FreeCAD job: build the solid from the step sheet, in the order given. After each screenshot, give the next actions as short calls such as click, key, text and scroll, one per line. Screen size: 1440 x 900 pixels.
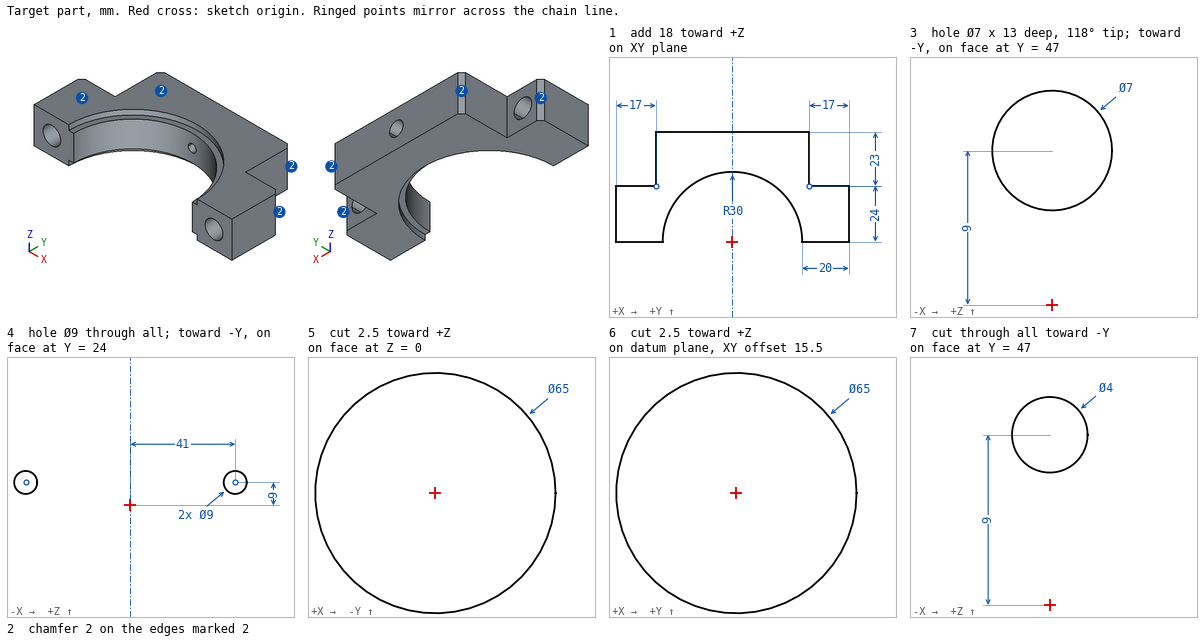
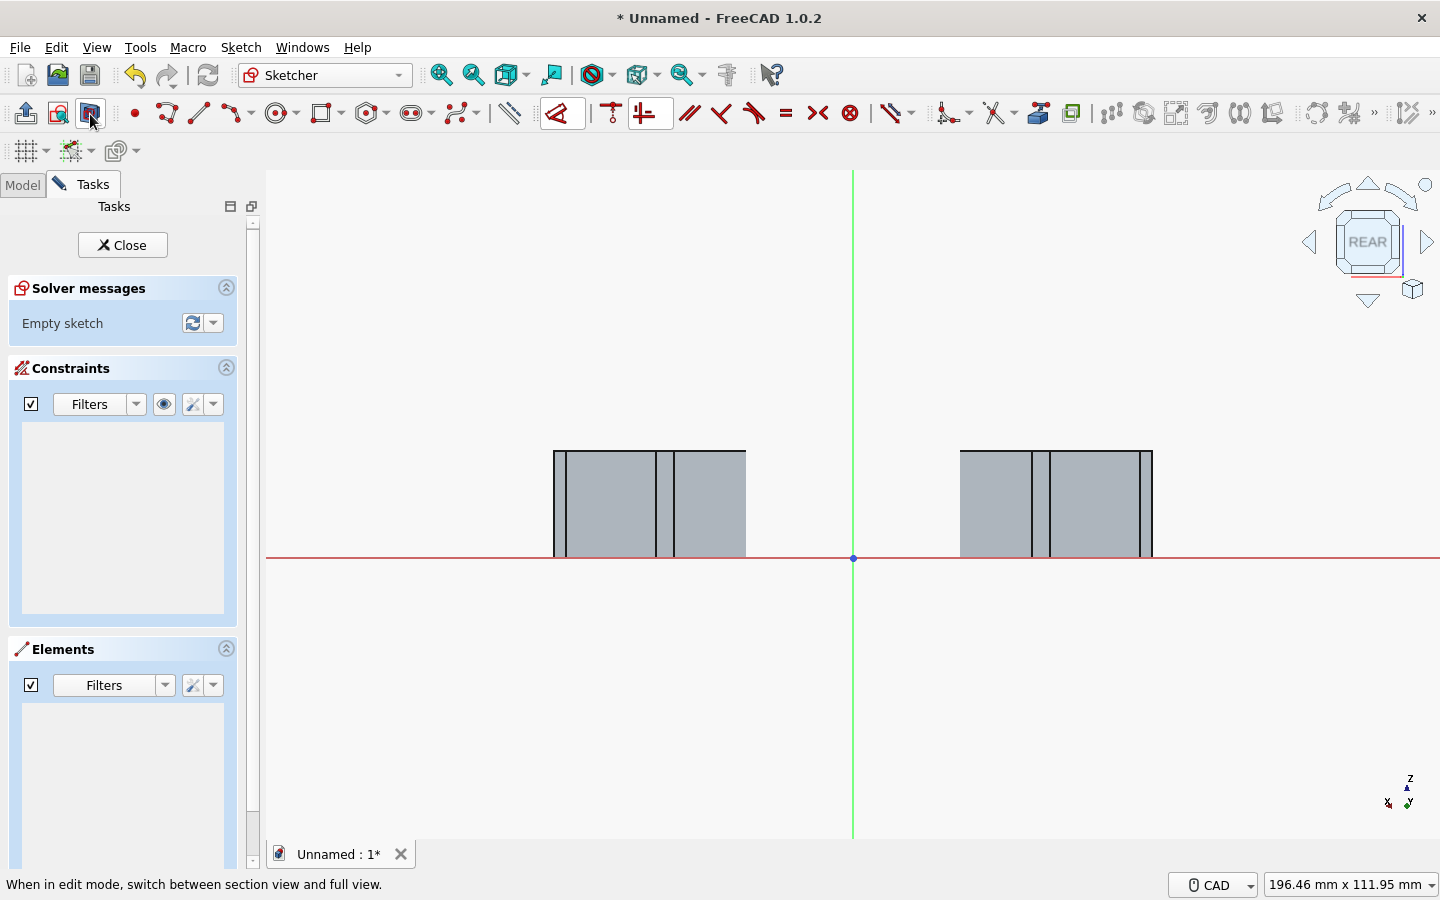
click(276, 114)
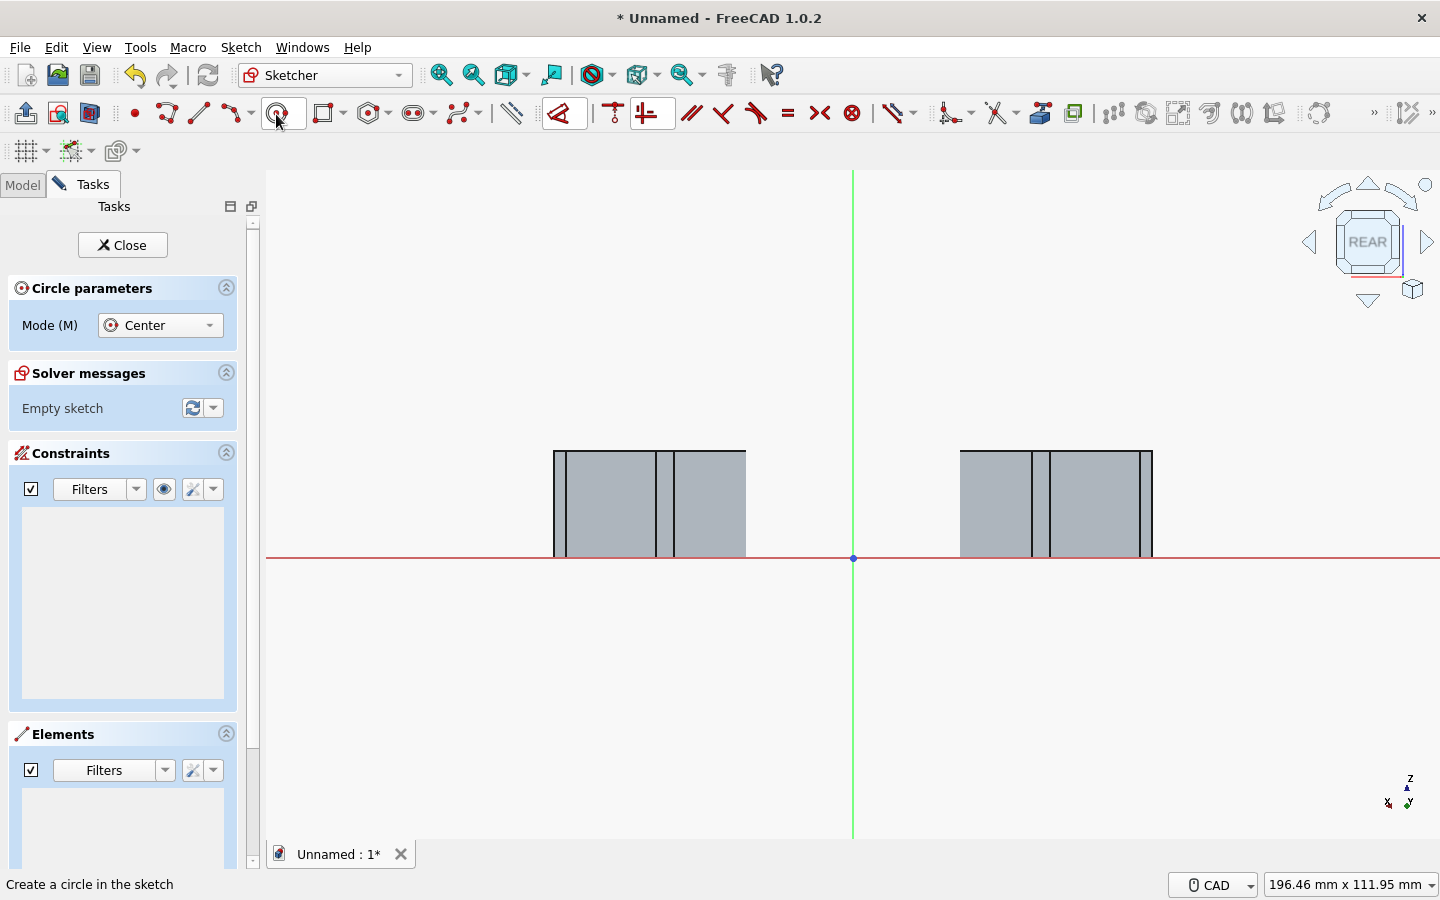
click(1098, 505)
click(1117, 485)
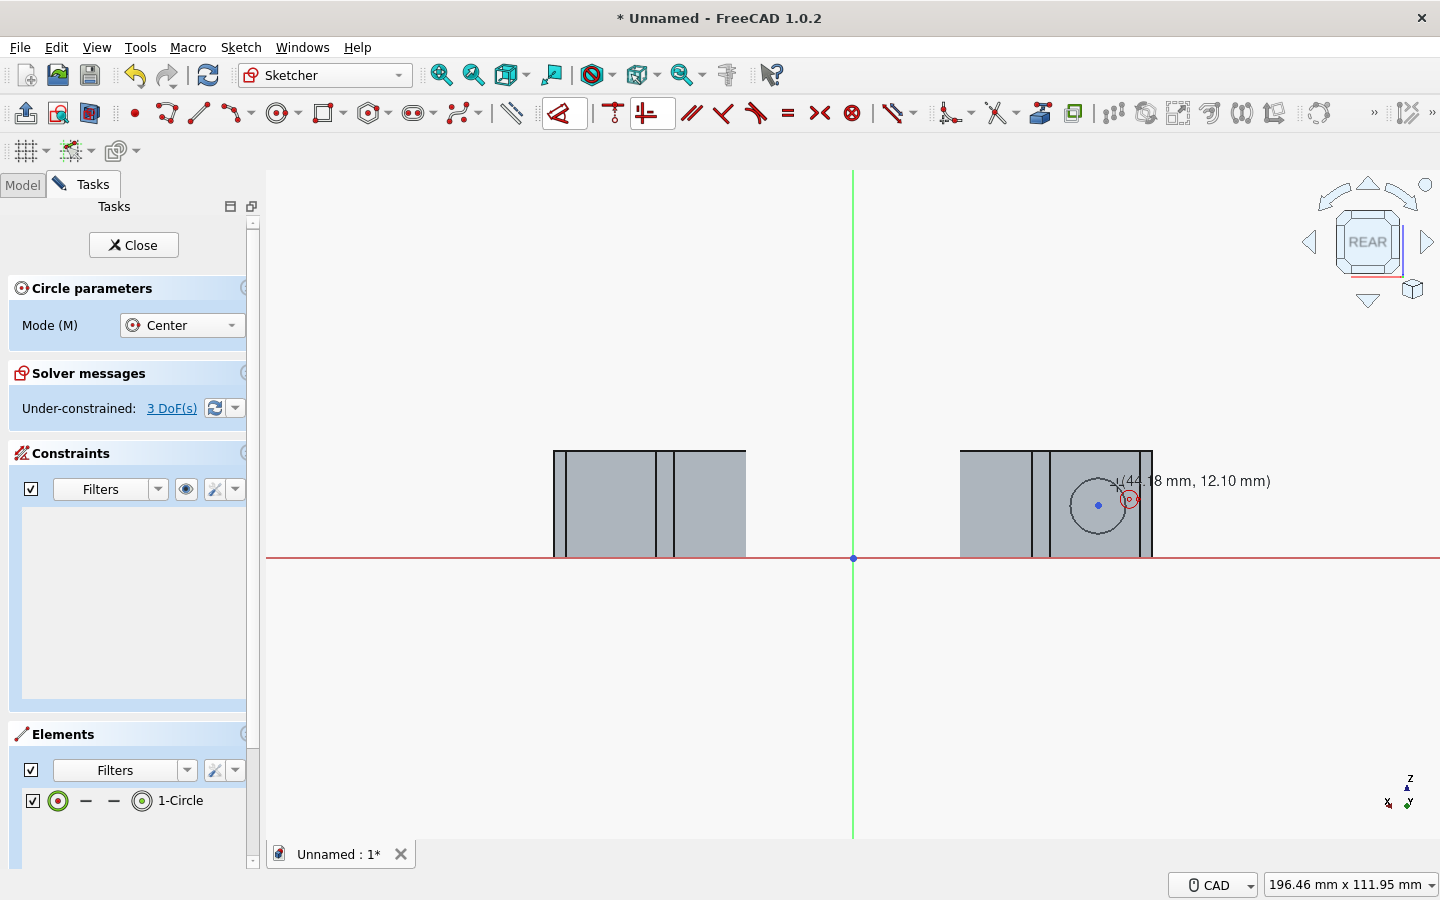
click(608, 505)
click(627, 485)
key(Escape)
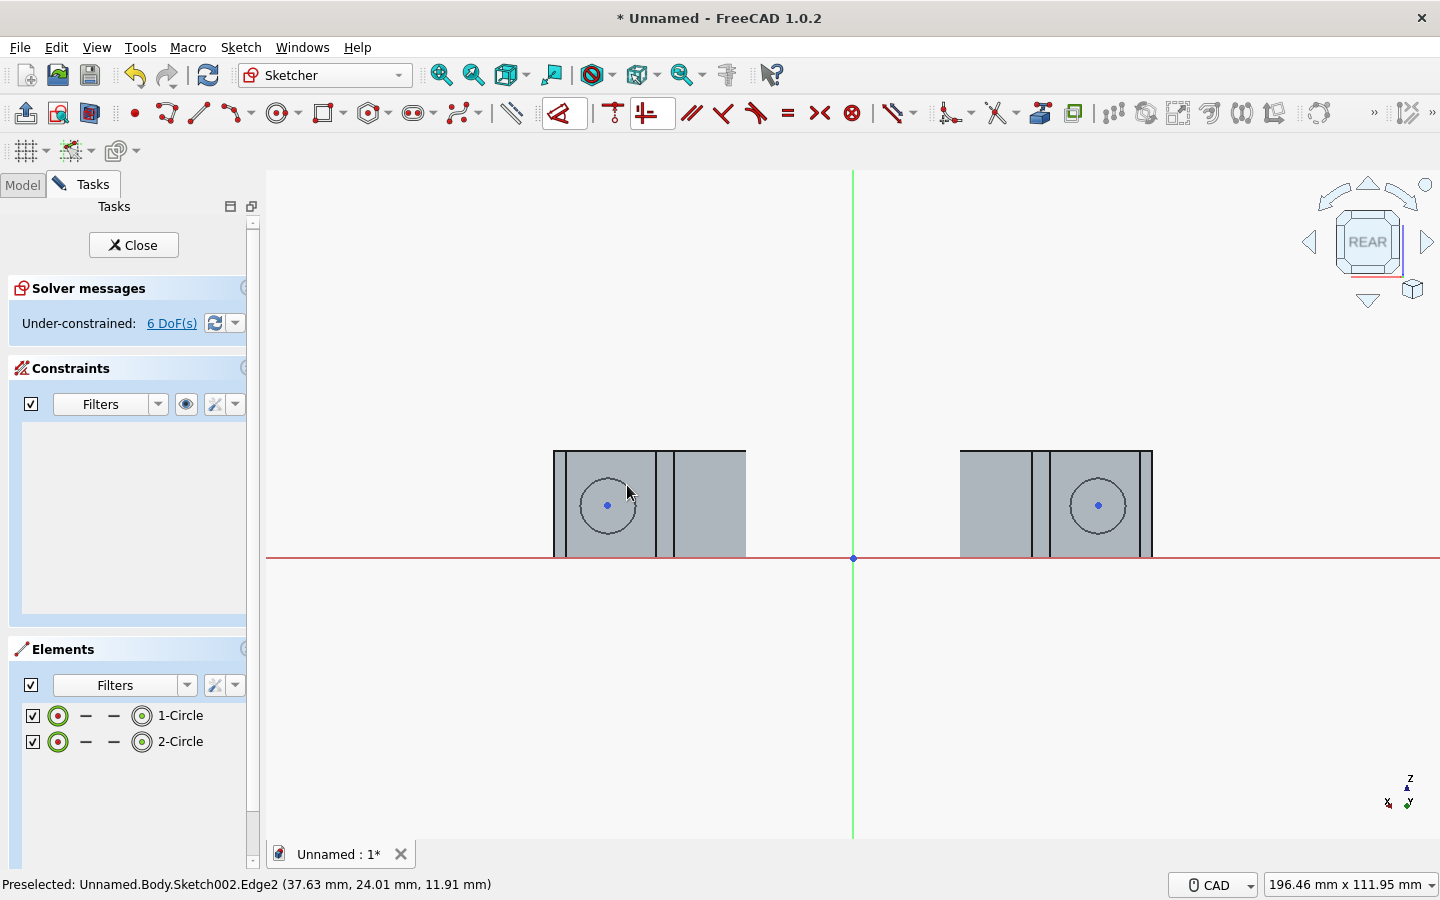
click(1117, 486)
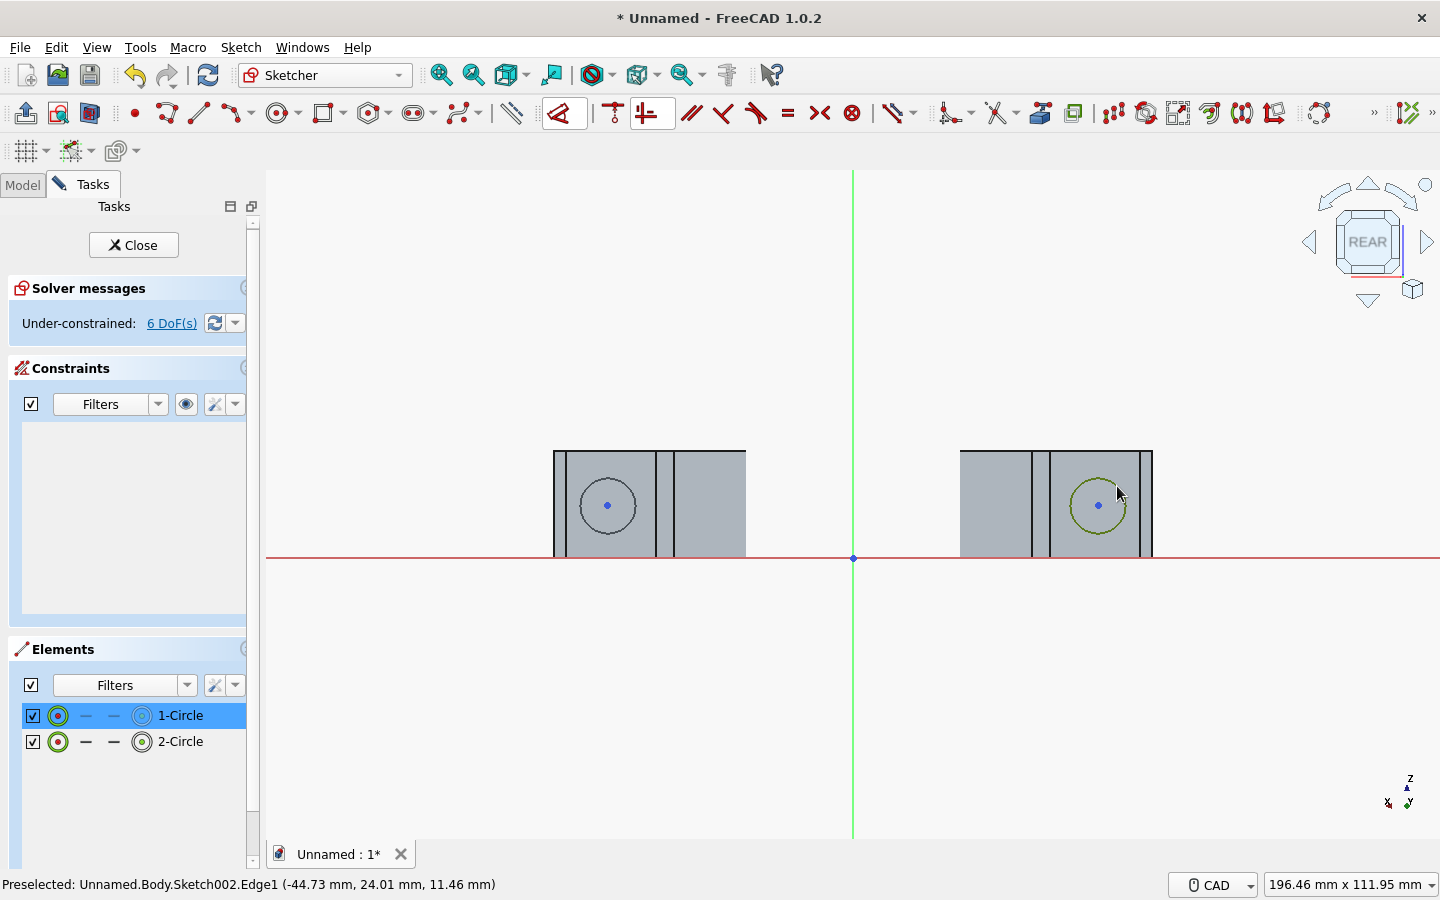
click(627, 486)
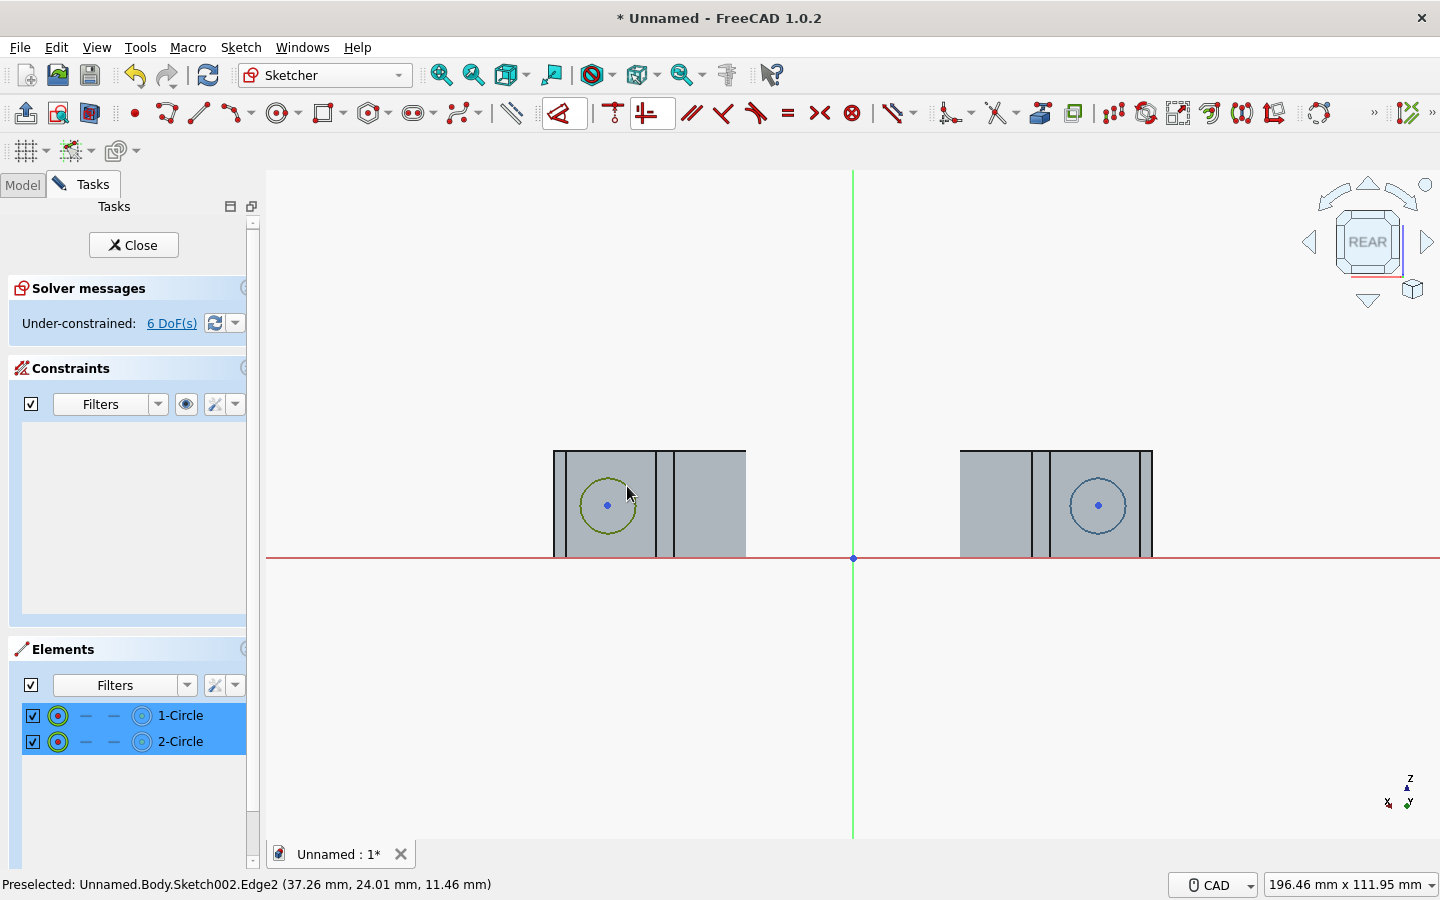
click(788, 114)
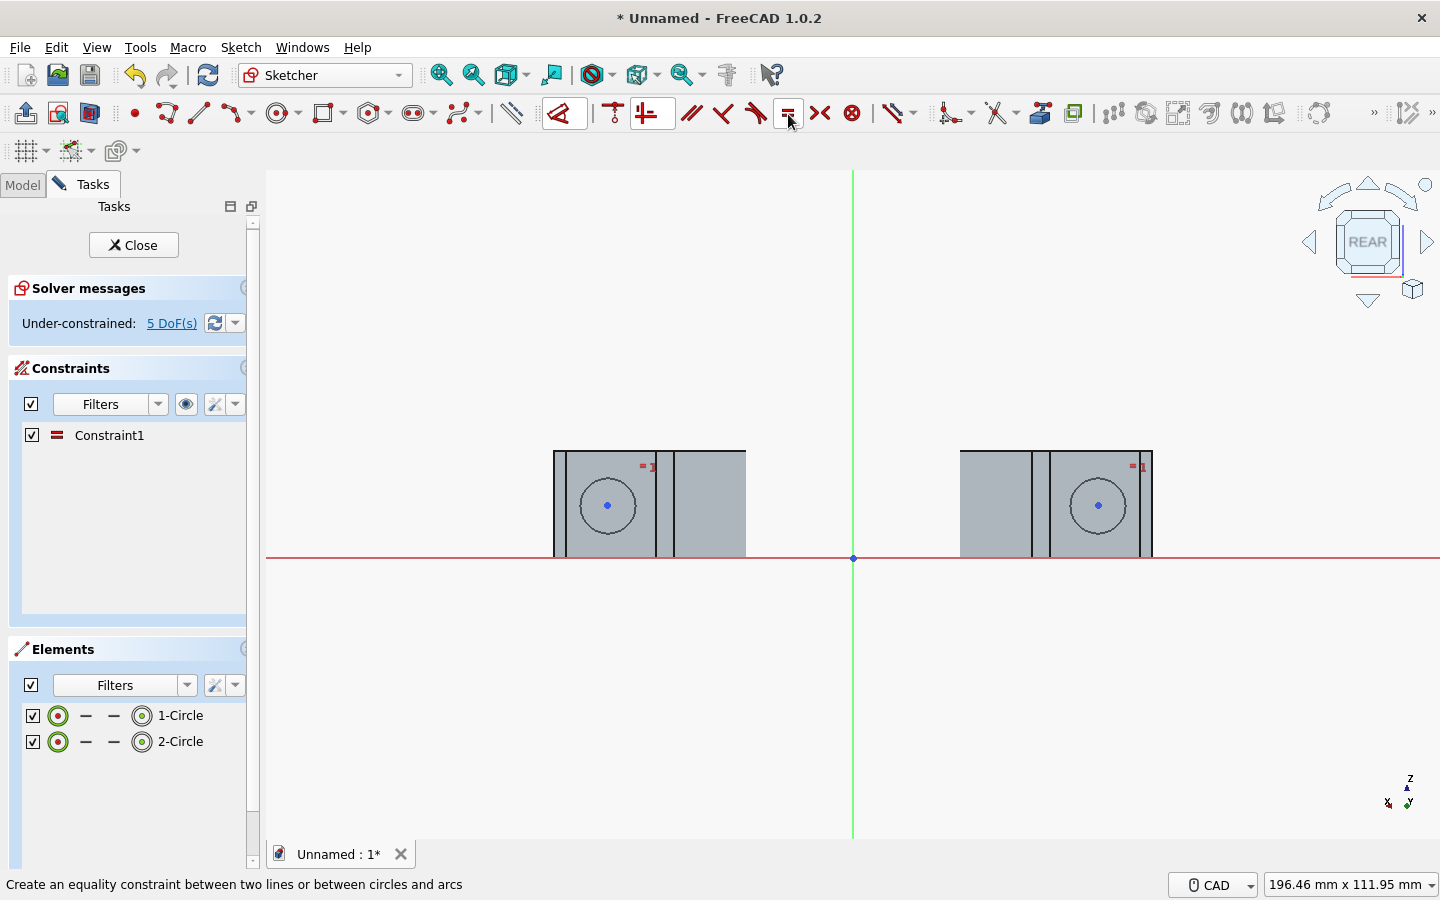
click(1098, 506)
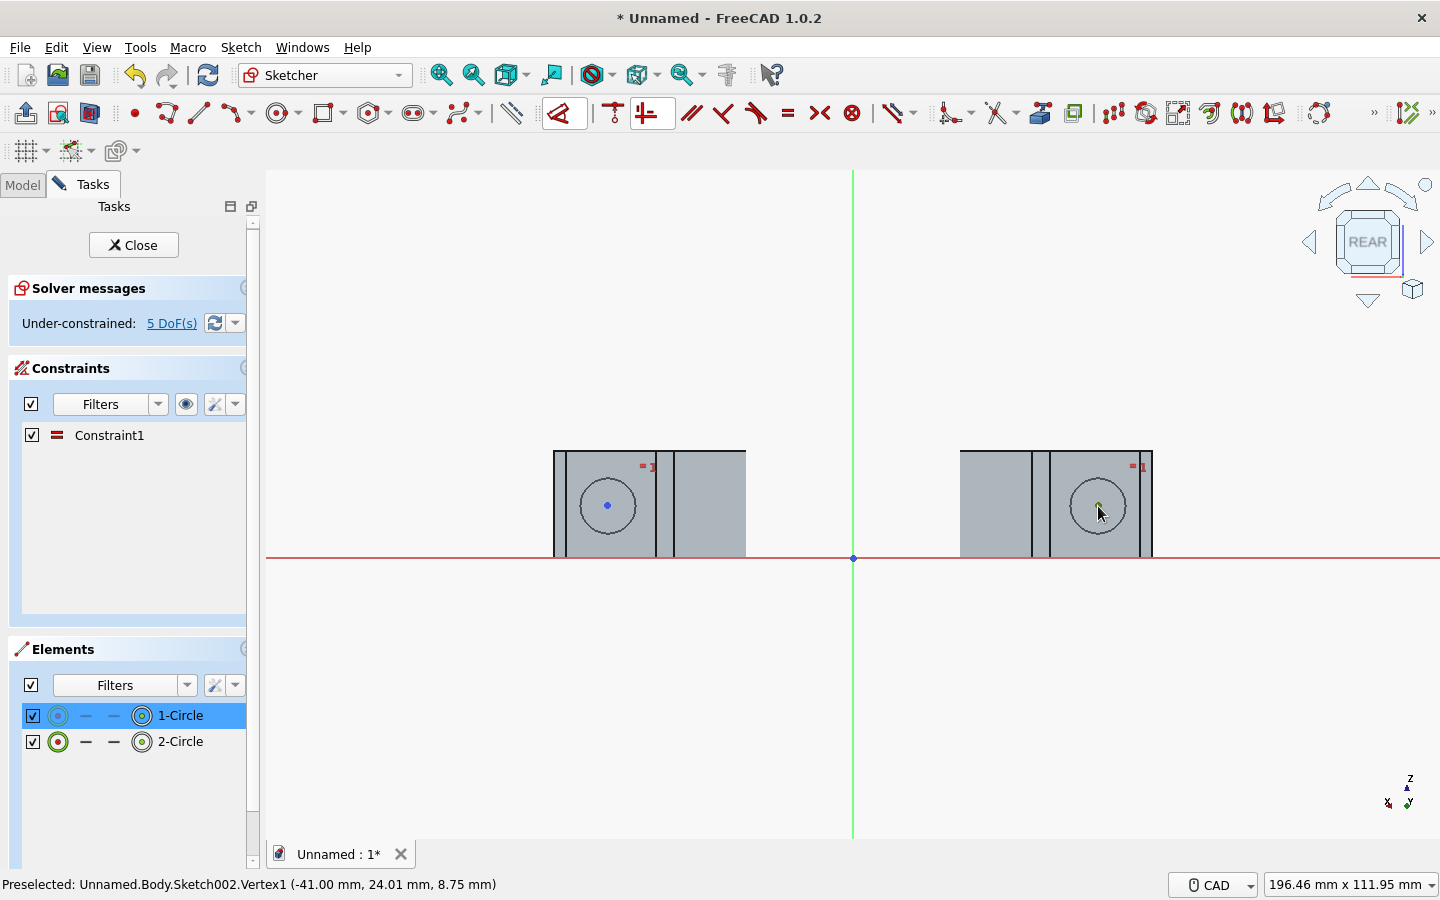
click(608, 506)